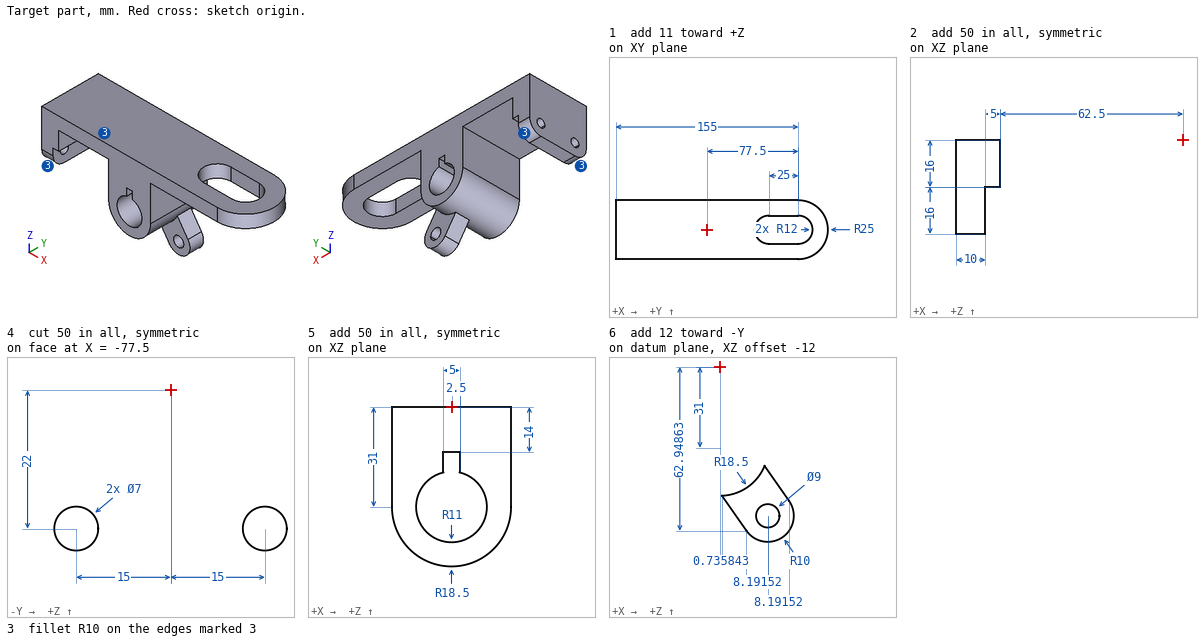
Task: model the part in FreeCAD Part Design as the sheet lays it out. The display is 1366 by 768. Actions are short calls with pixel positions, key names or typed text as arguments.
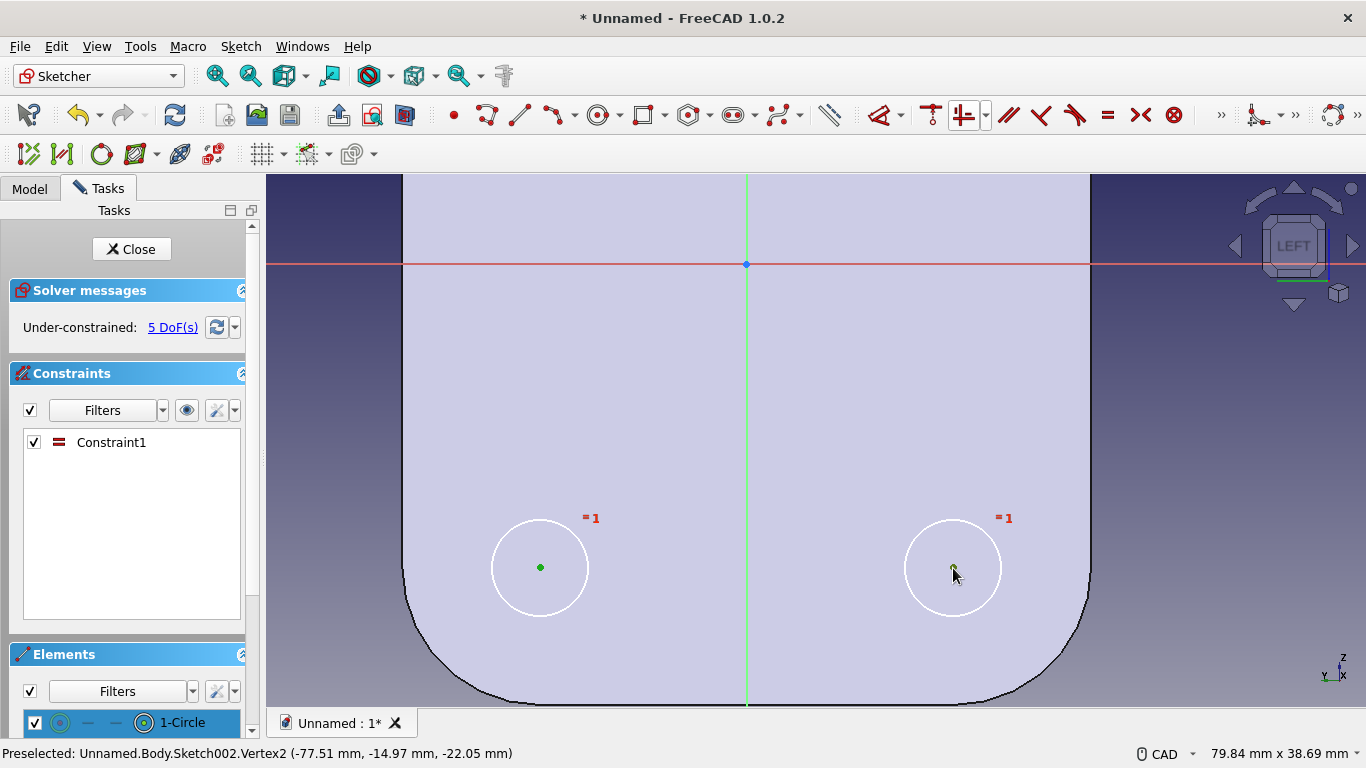
key(h)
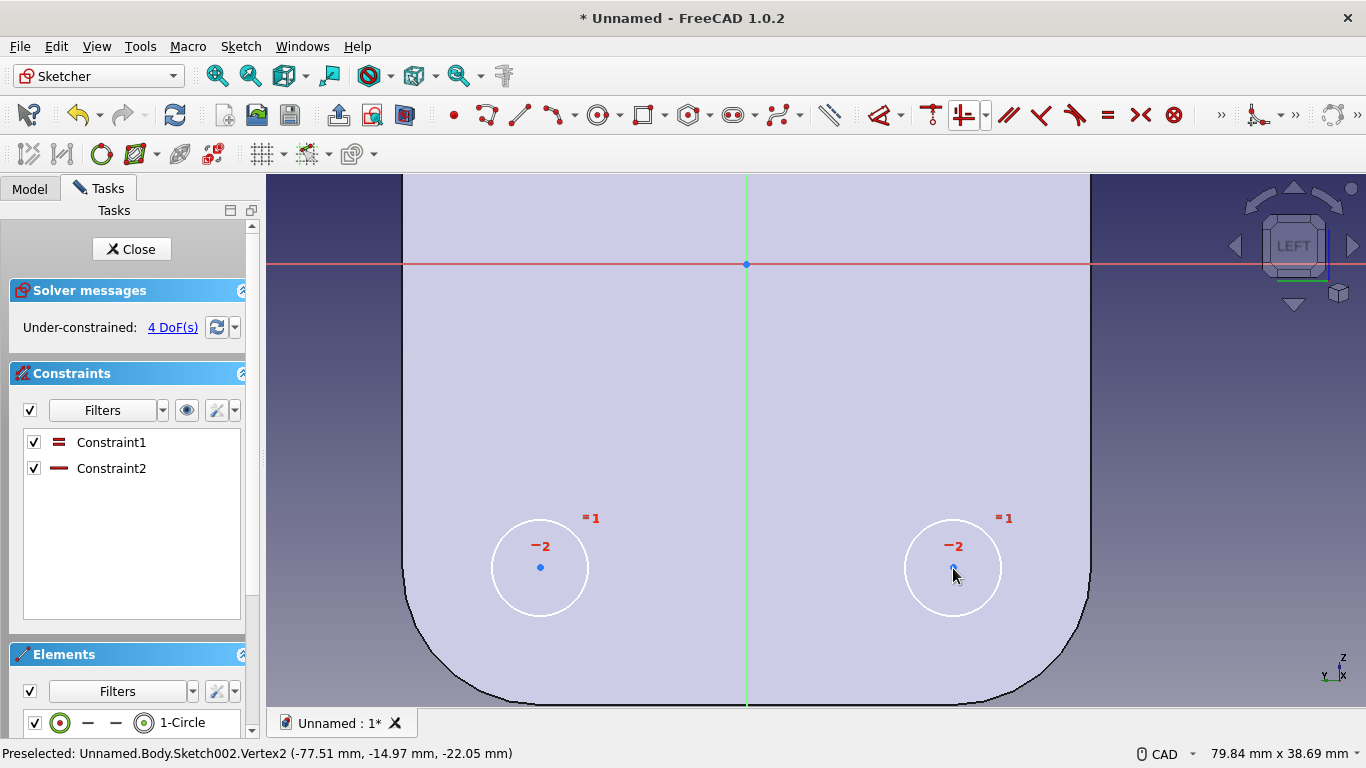
click(878, 116)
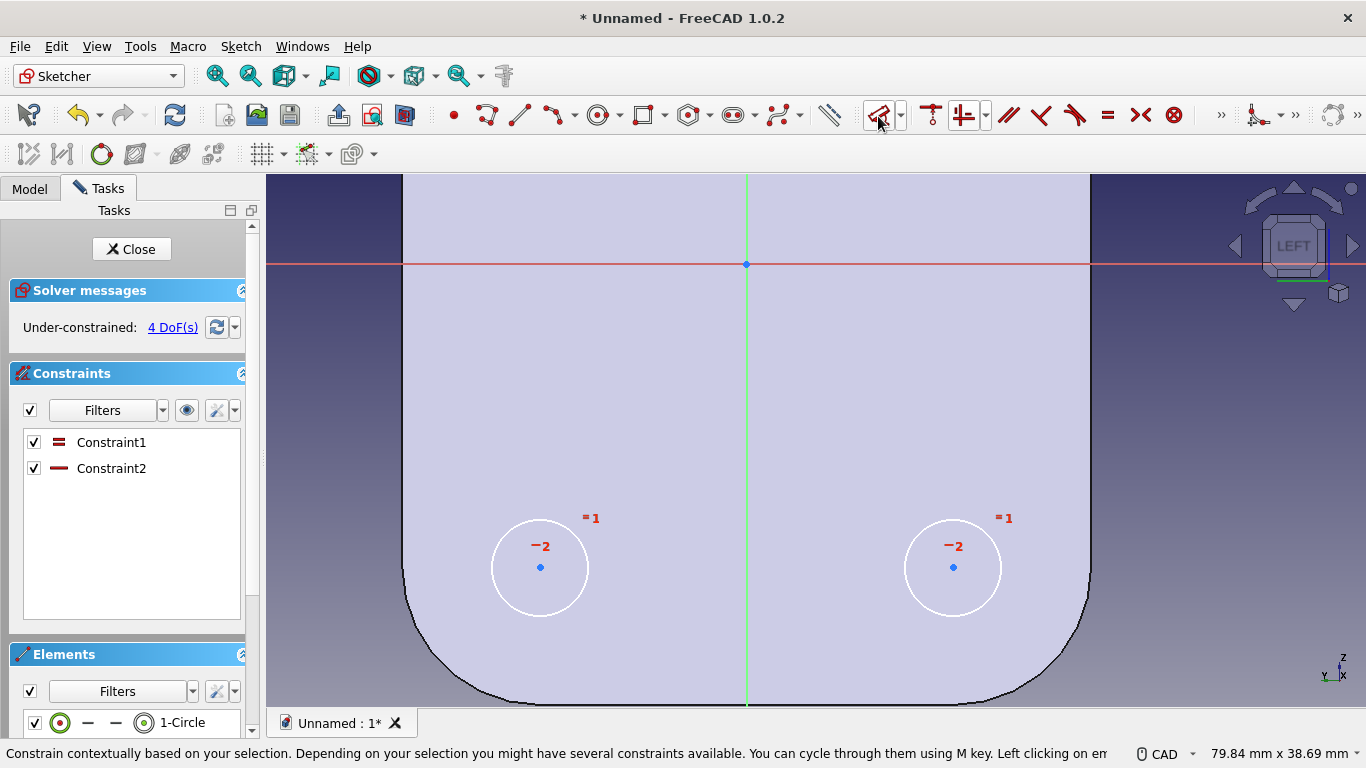
click(574, 534)
click(597, 511)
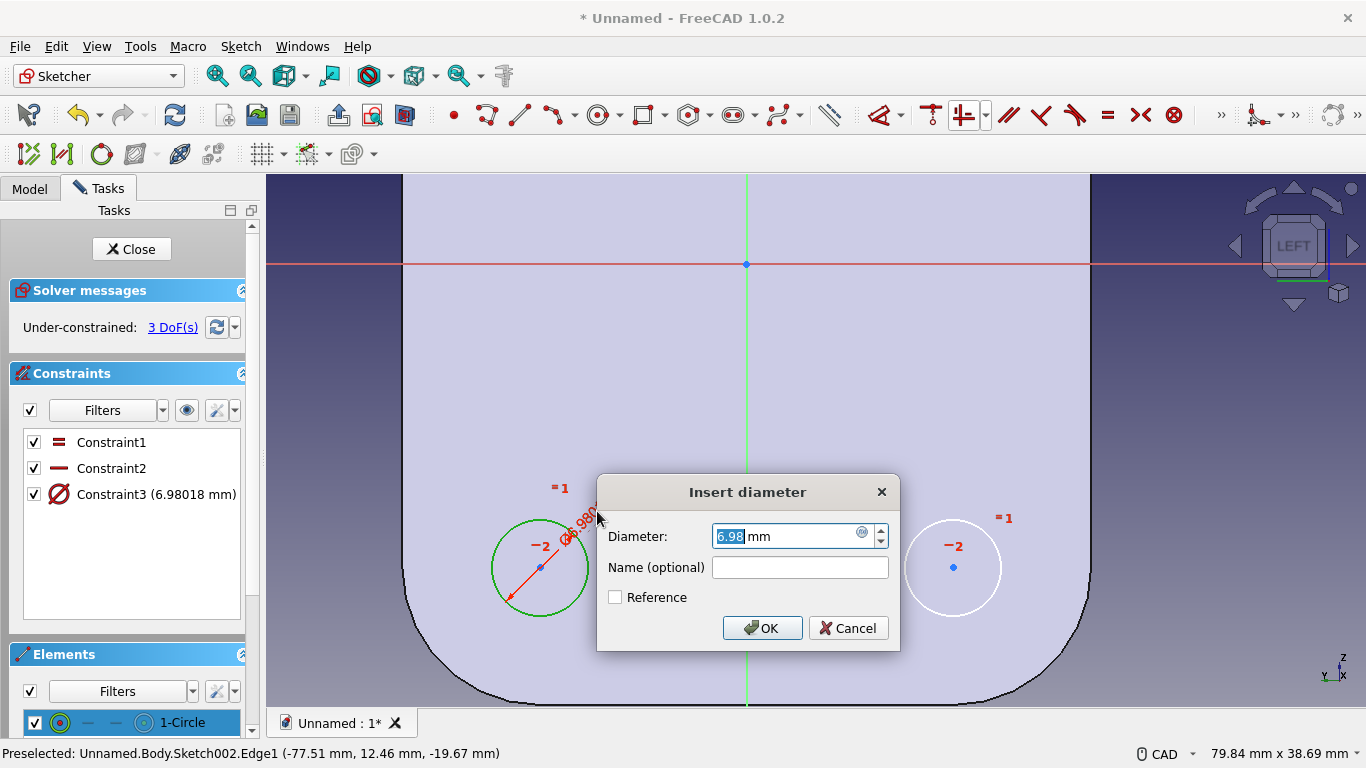
text(7)
key(Return)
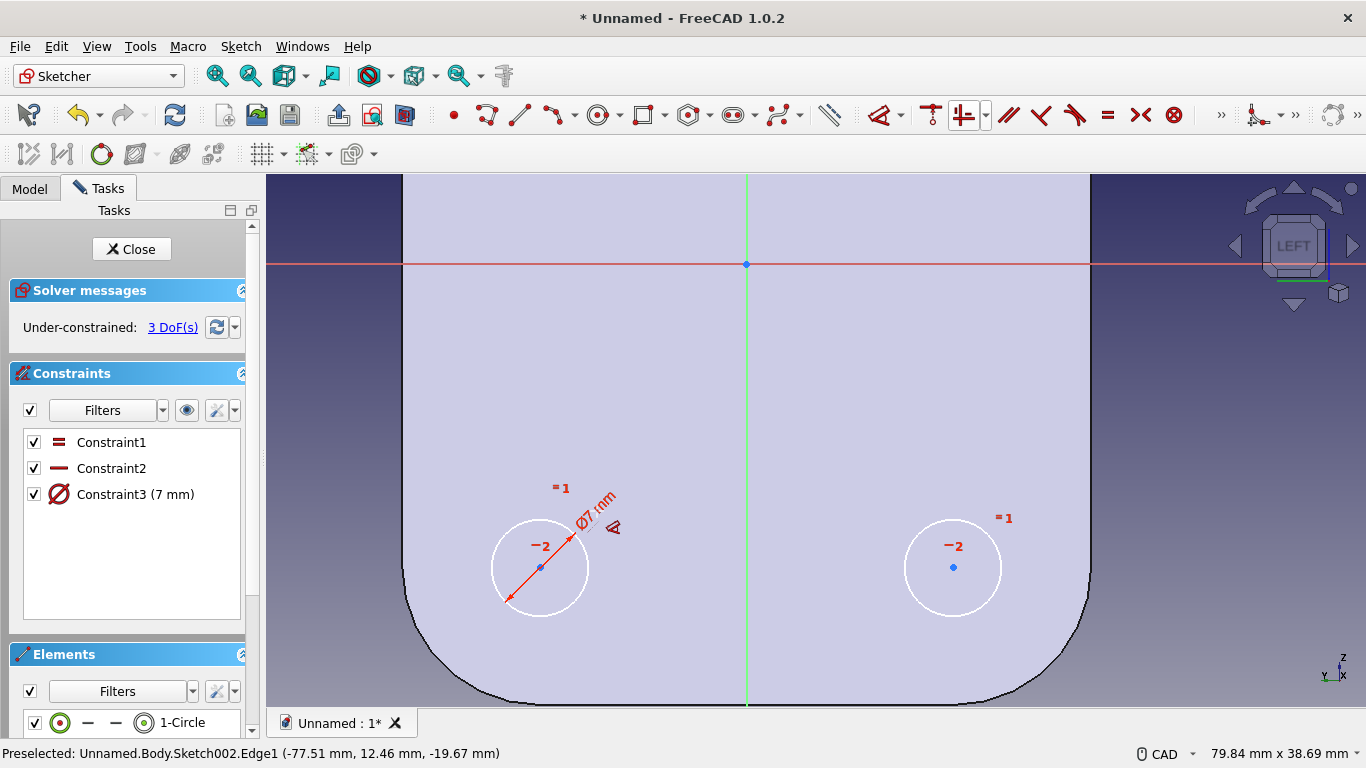
click(540, 568)
click(643, 230)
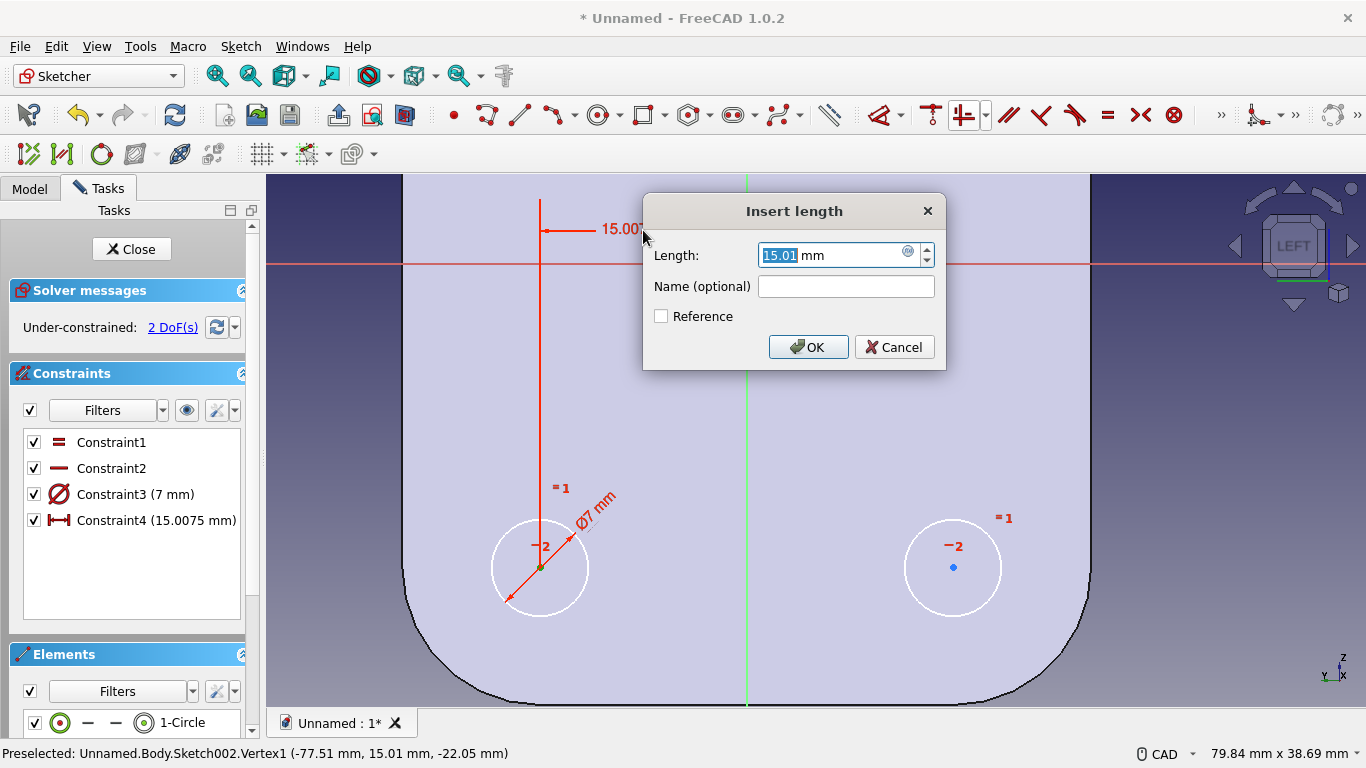
text(15)
key(Return)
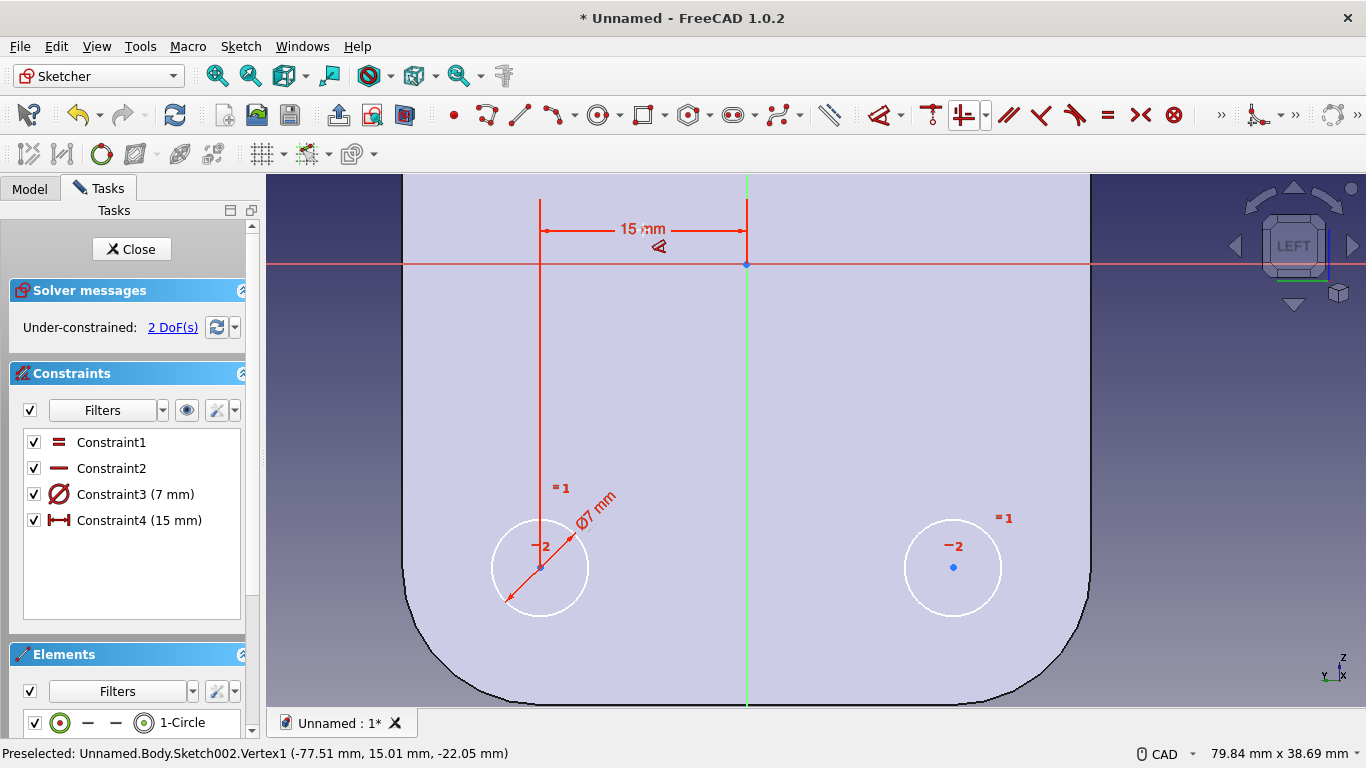
click(540, 568)
click(506, 416)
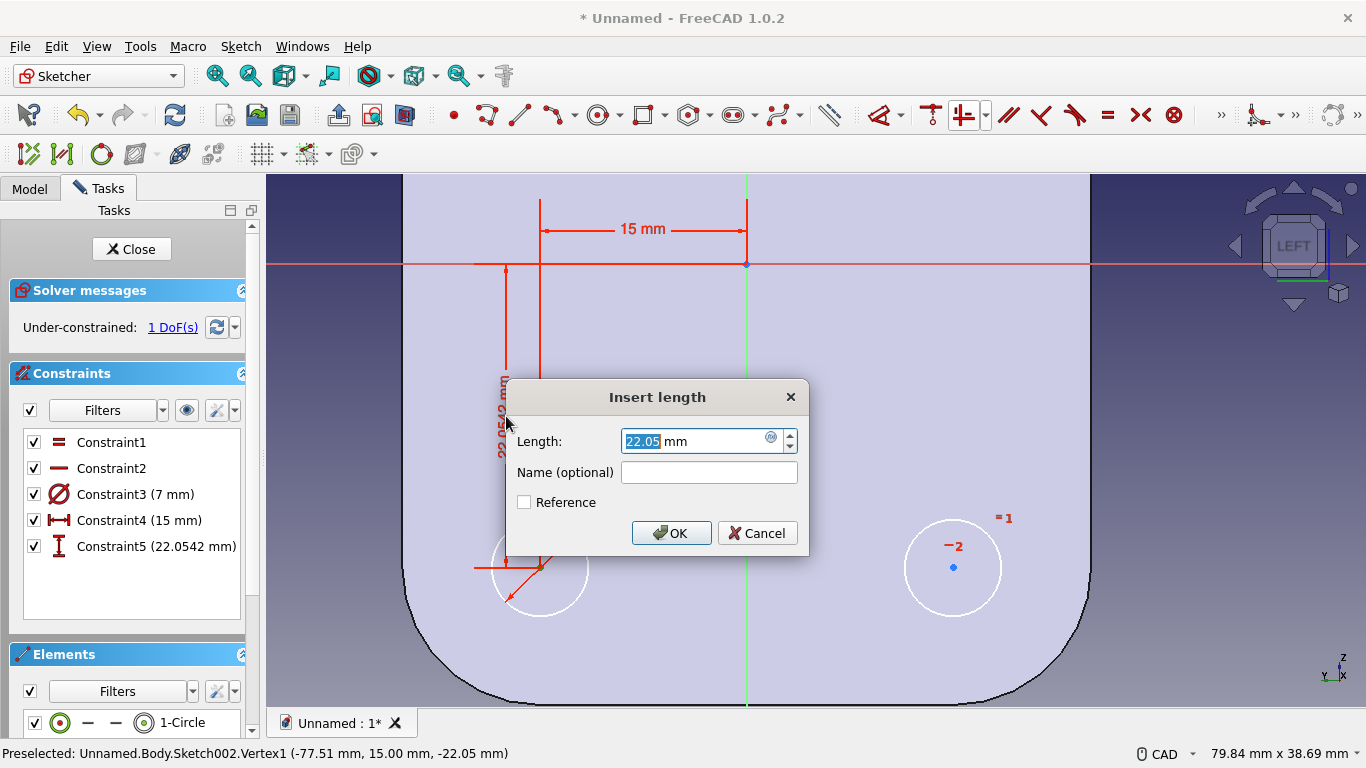
text(22)
key(Return)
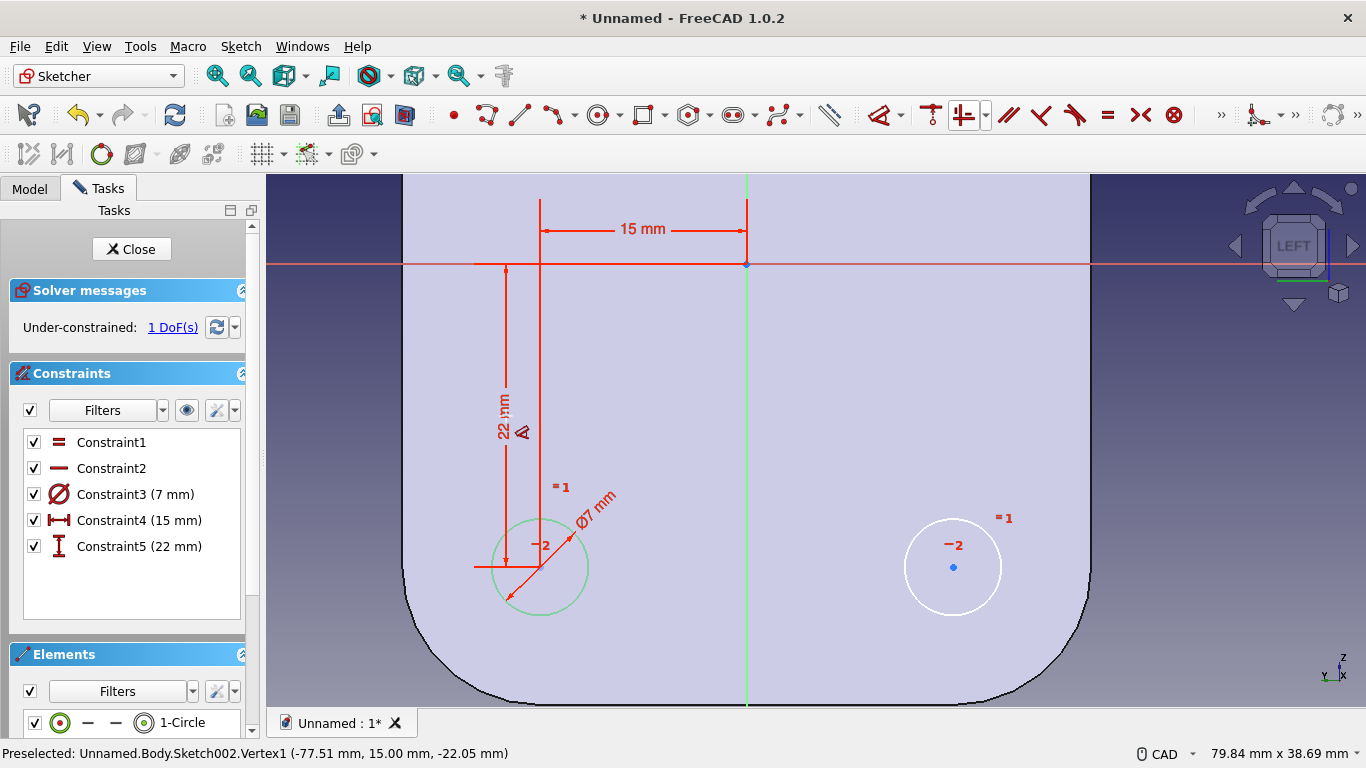
click(953, 567)
click(850, 230)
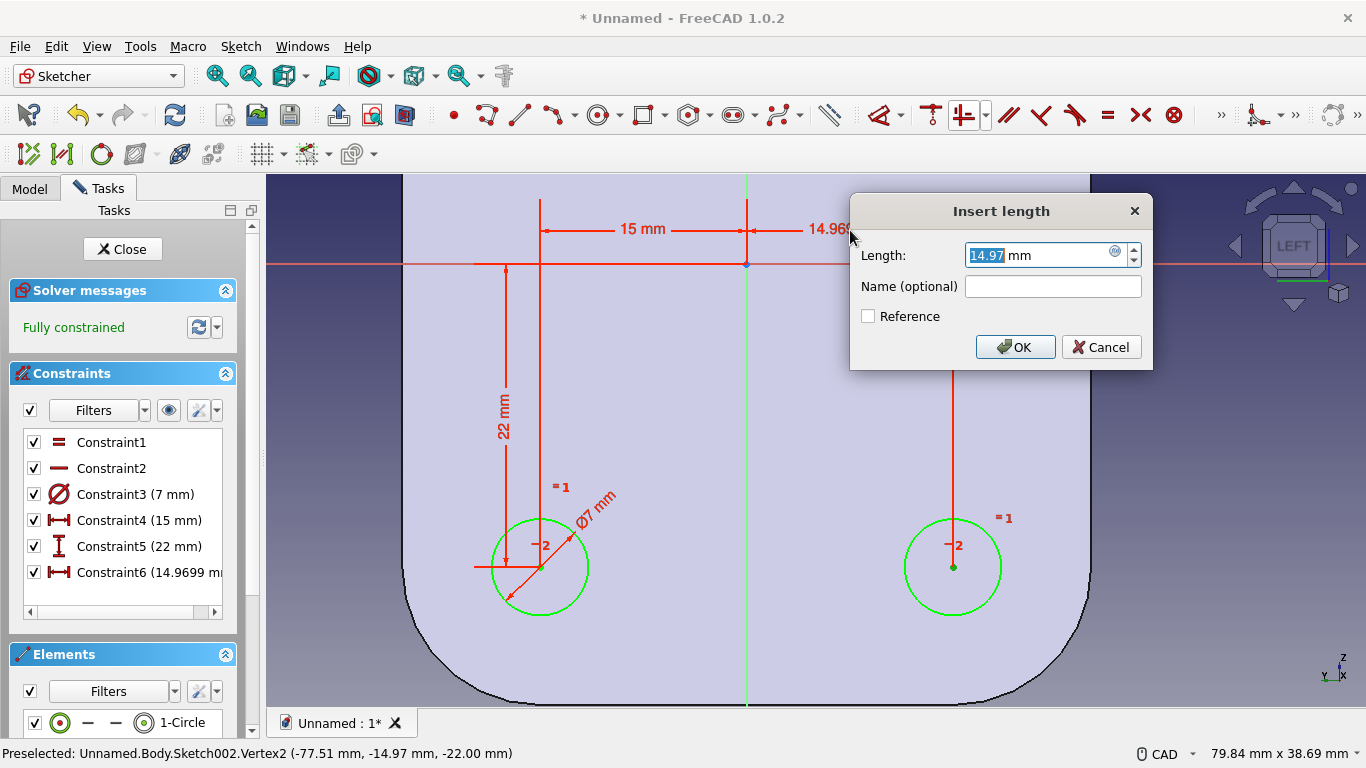
text(15)
key(Return)
key(Escape)